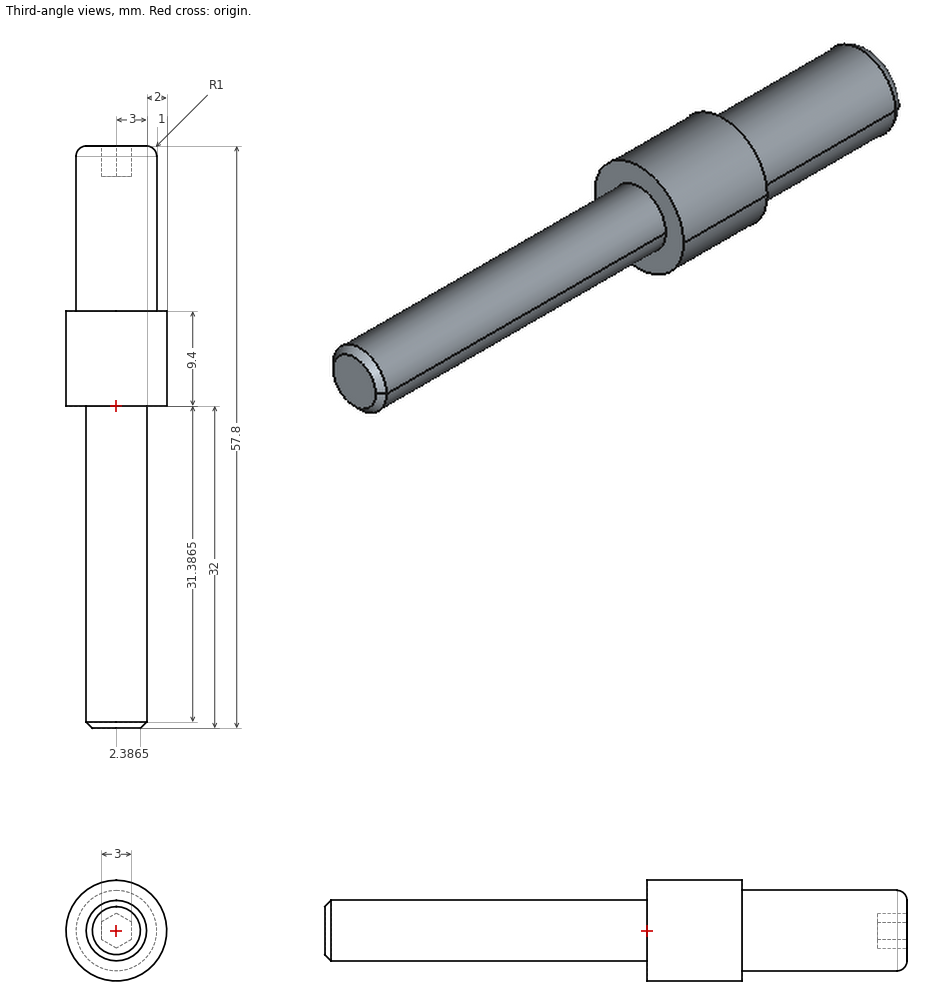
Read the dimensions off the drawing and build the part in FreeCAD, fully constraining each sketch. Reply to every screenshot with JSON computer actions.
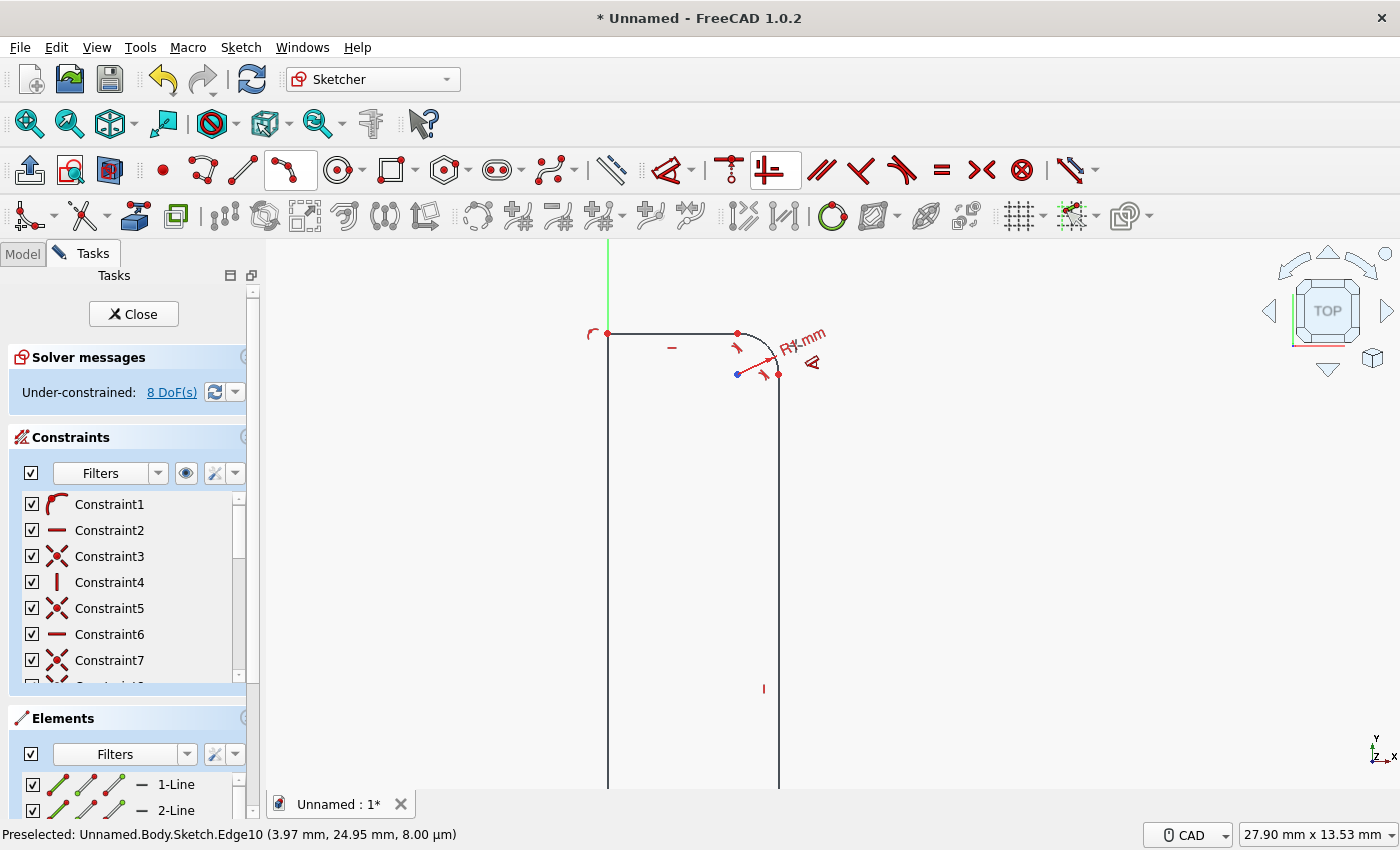
{"action": "left_click", "coordinate": [699, 334]}
{"action": "left_click", "coordinate": [673, 300]}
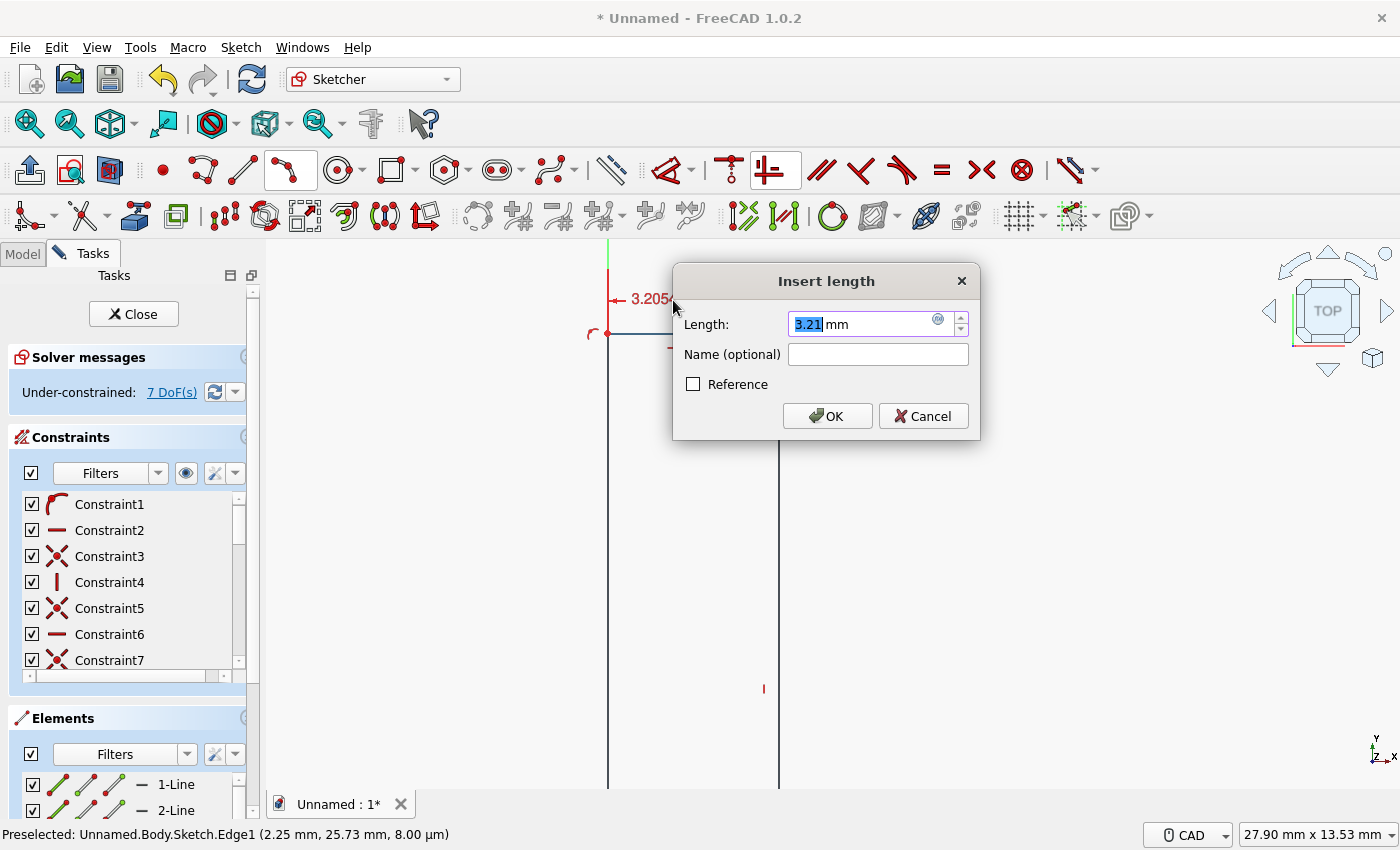
{"action": "type", "text": "3"}
{"action": "key", "text": "Return"}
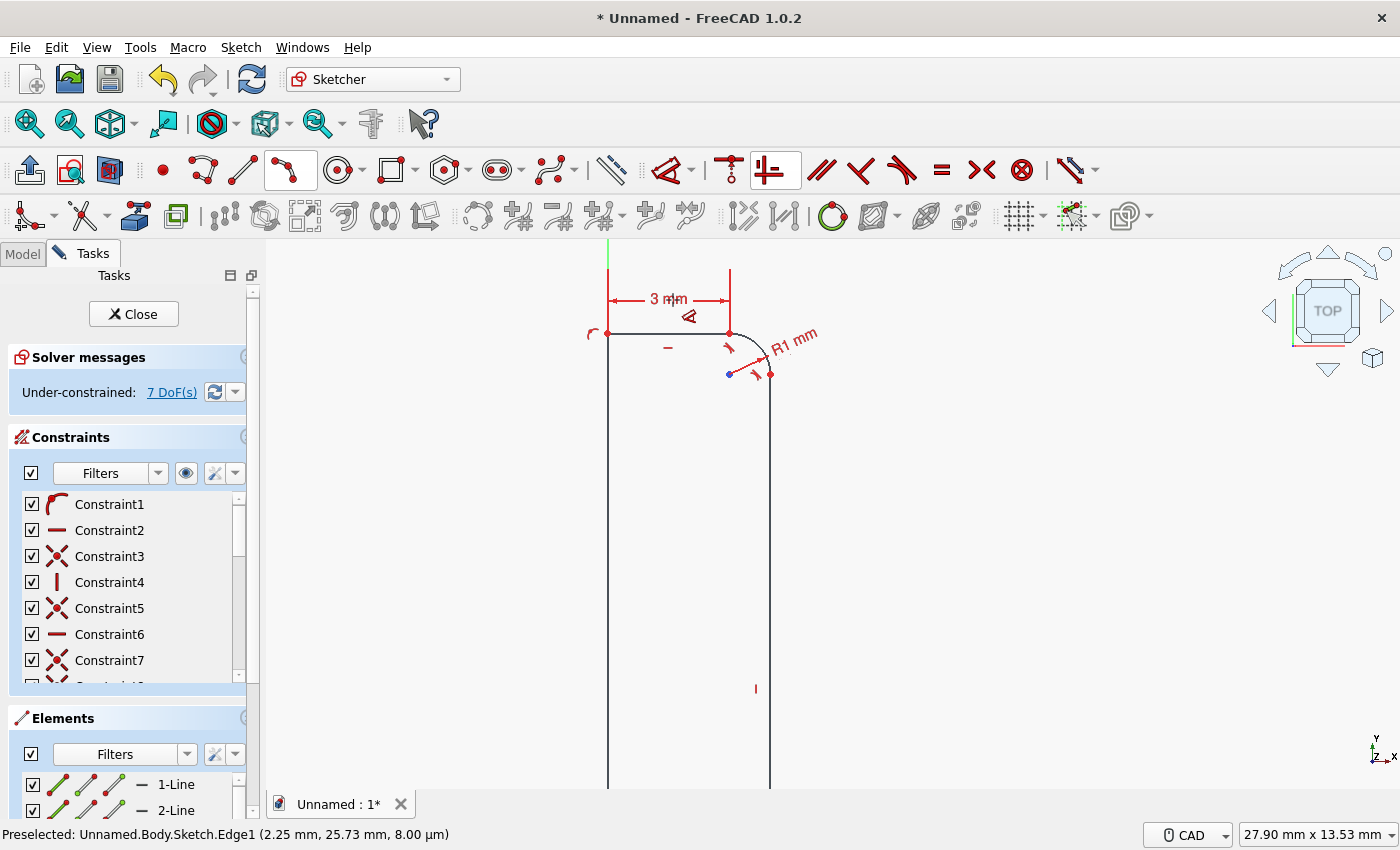
{"action": "scroll", "coordinate": [773, 359], "scroll_direction": "down", "scroll_amount": 10}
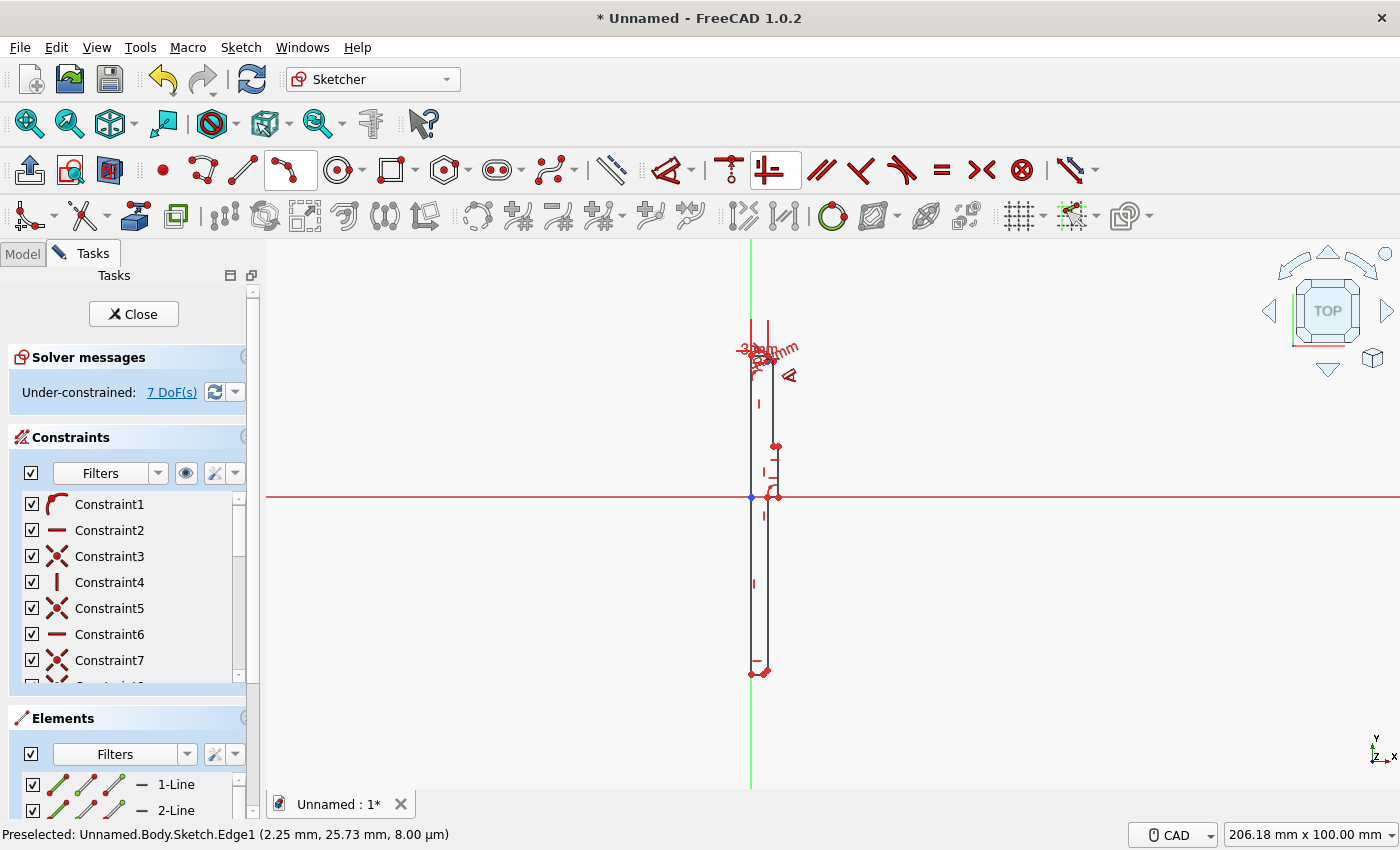
{"action": "scroll", "coordinate": [771, 497], "scroll_direction": "up", "scroll_amount": 8}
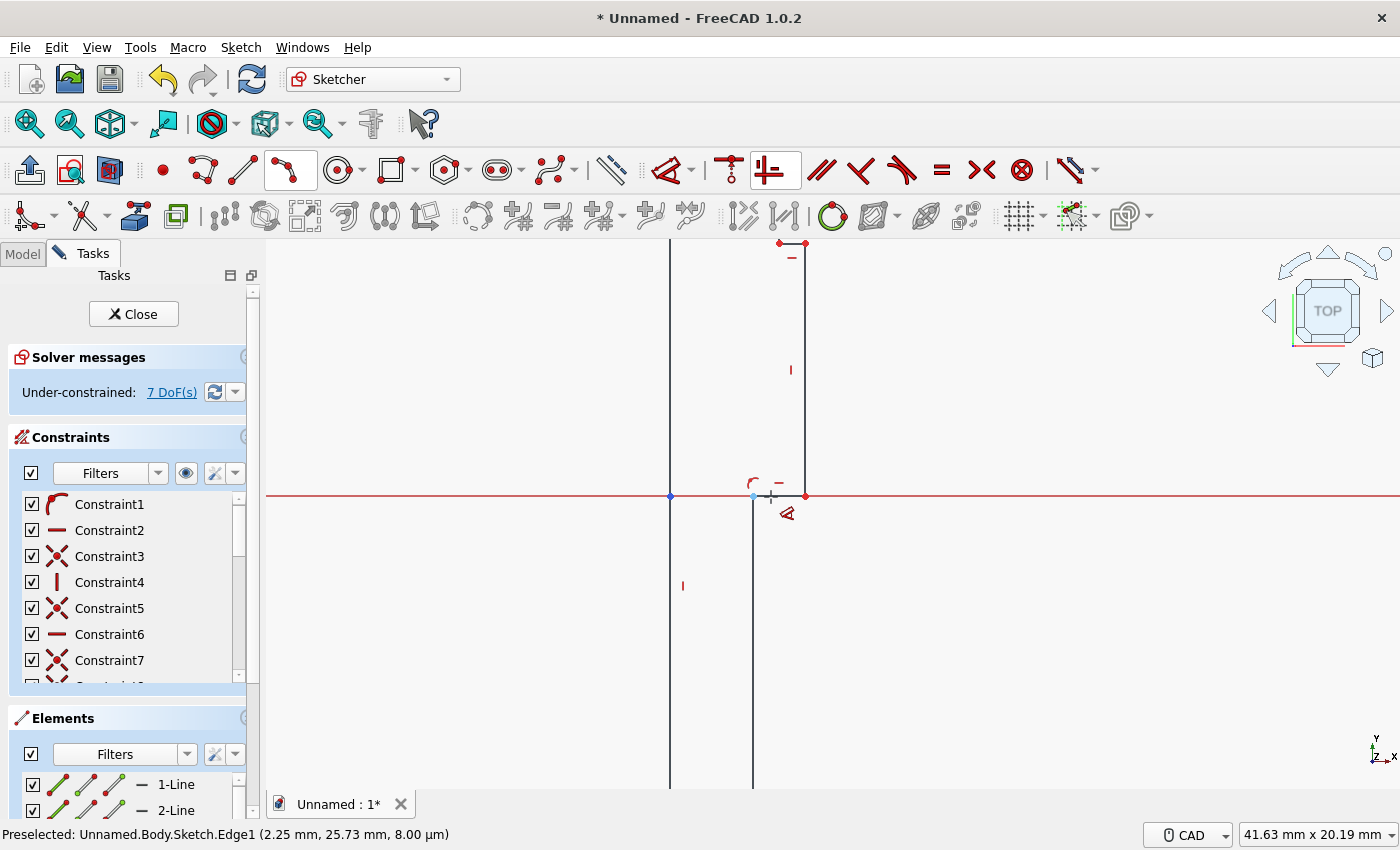
{"action": "left_click", "coordinate": [769, 496]}
{"action": "left_click", "coordinate": [779, 462]}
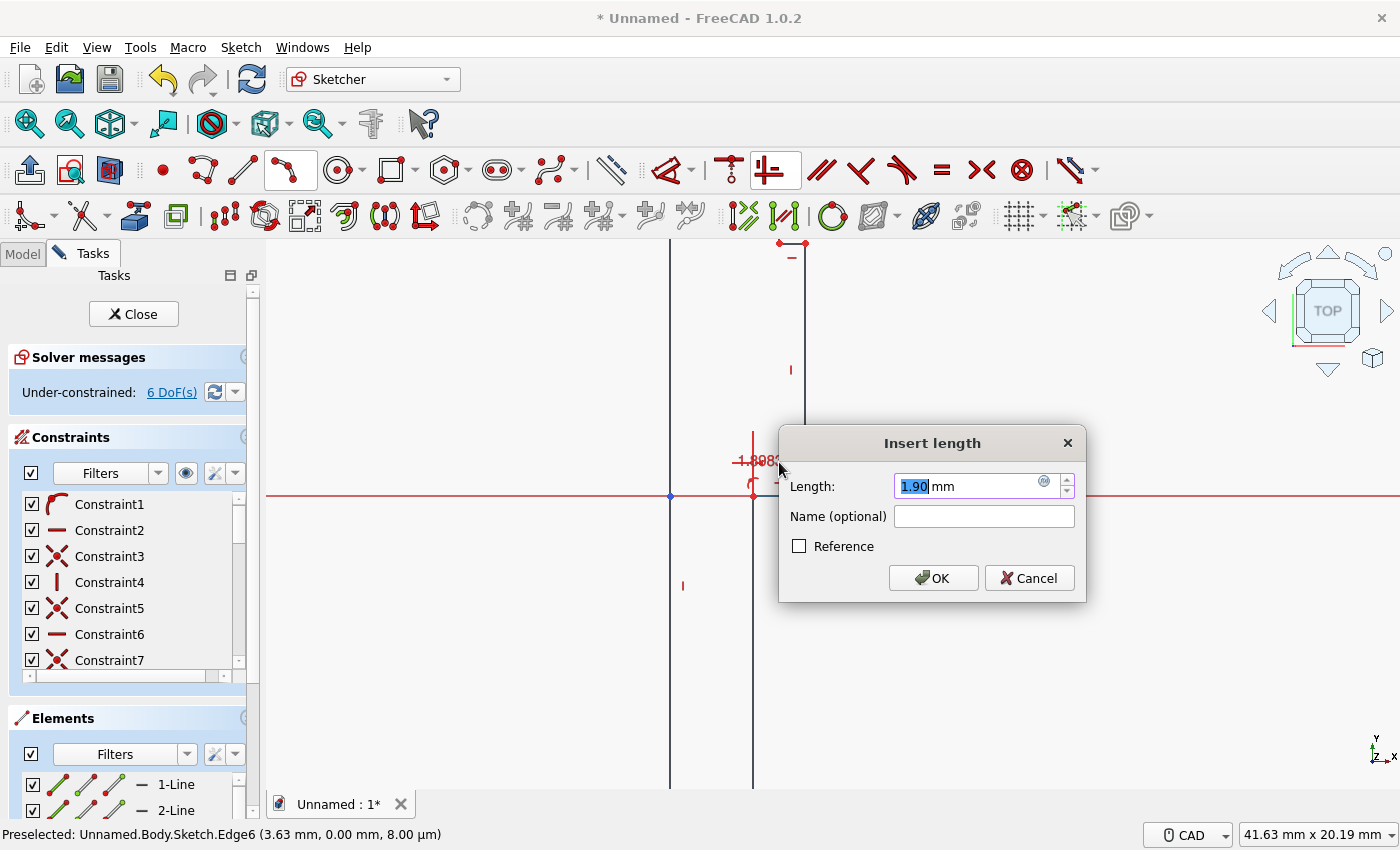
{"action": "type", "text": "2"}
{"action": "key", "text": "Return"}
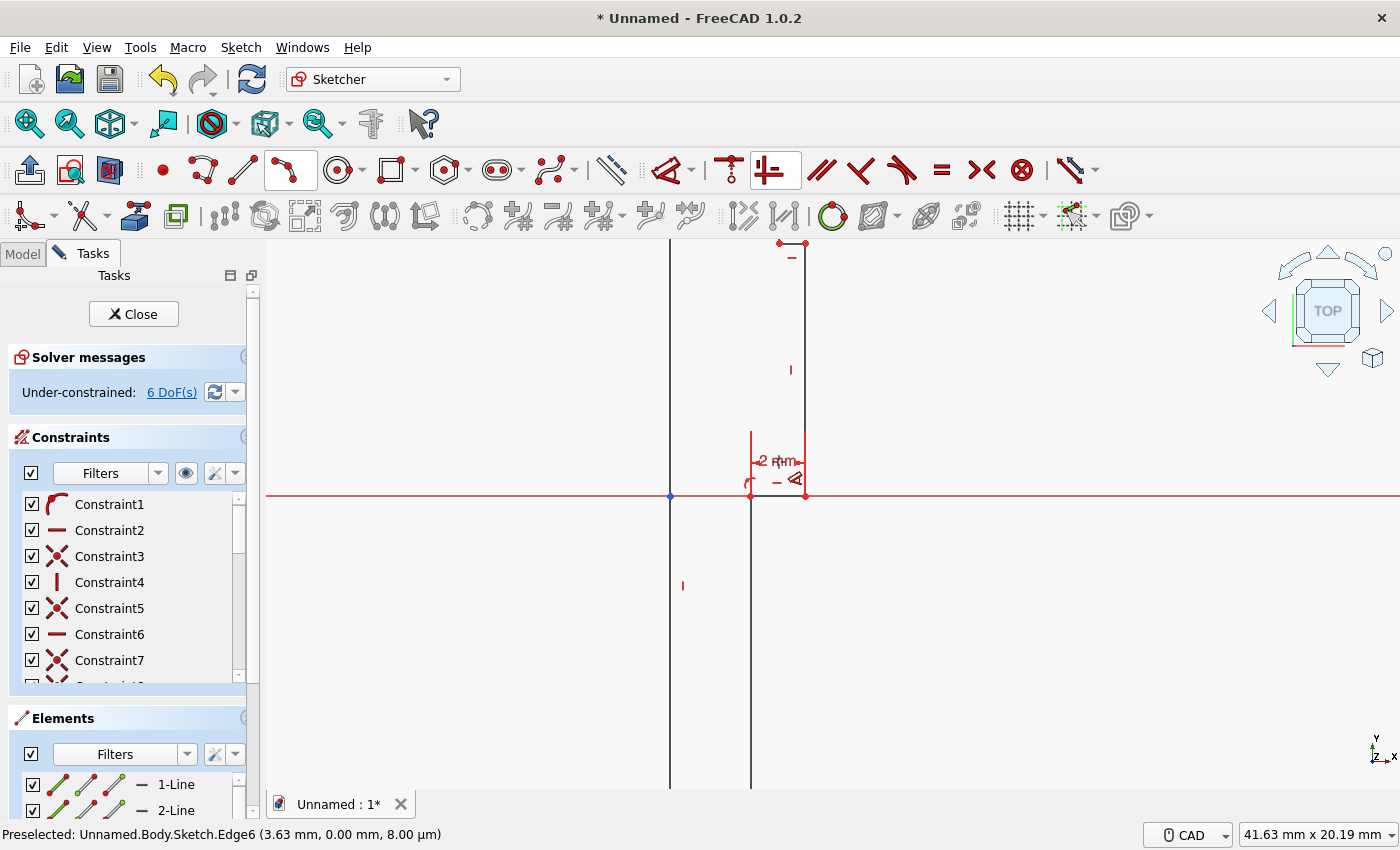
{"action": "scroll", "coordinate": [771, 497], "scroll_direction": "down", "scroll_amount": 8}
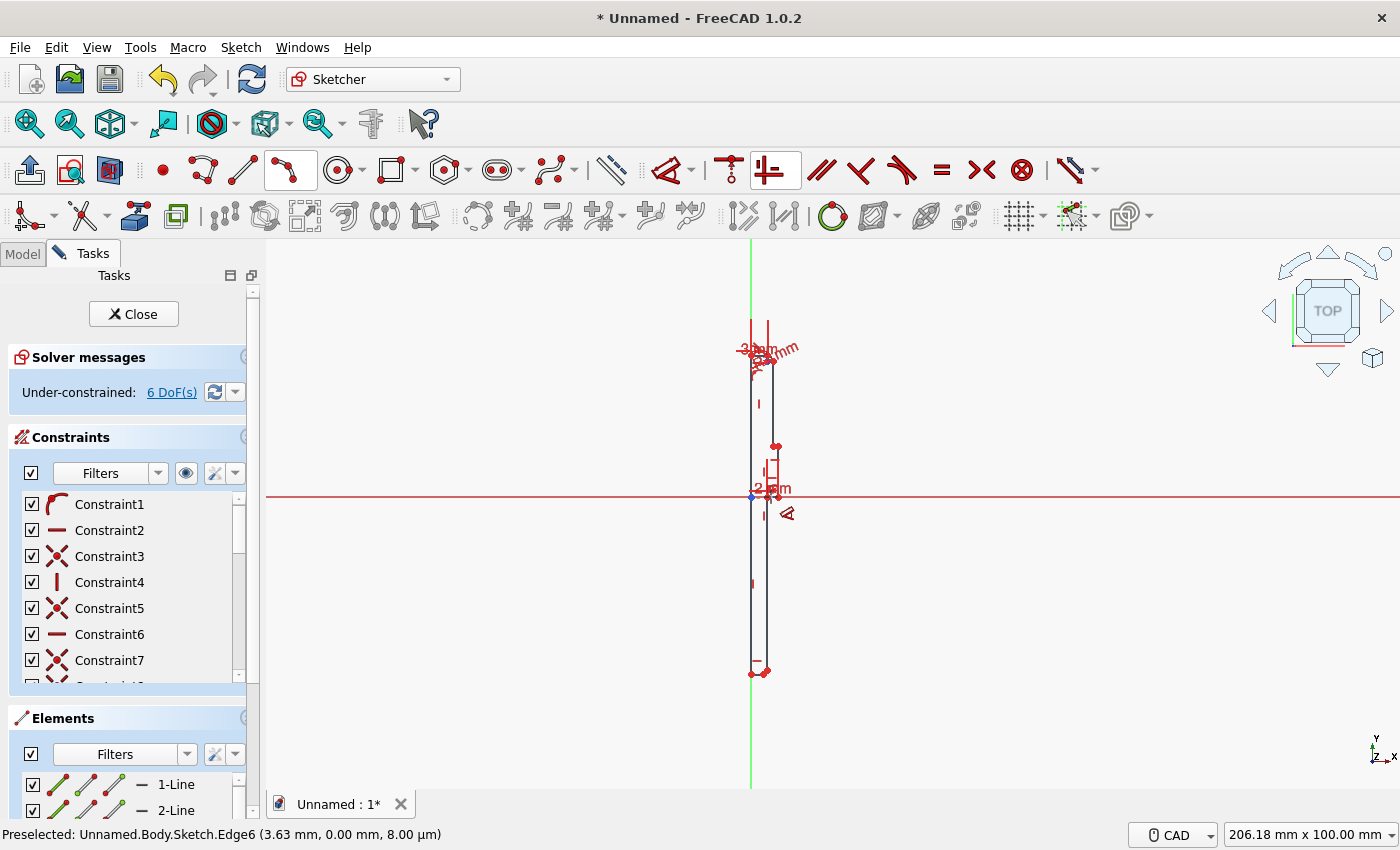
{"action": "scroll", "coordinate": [776, 446], "scroll_direction": "up", "scroll_amount": 10}